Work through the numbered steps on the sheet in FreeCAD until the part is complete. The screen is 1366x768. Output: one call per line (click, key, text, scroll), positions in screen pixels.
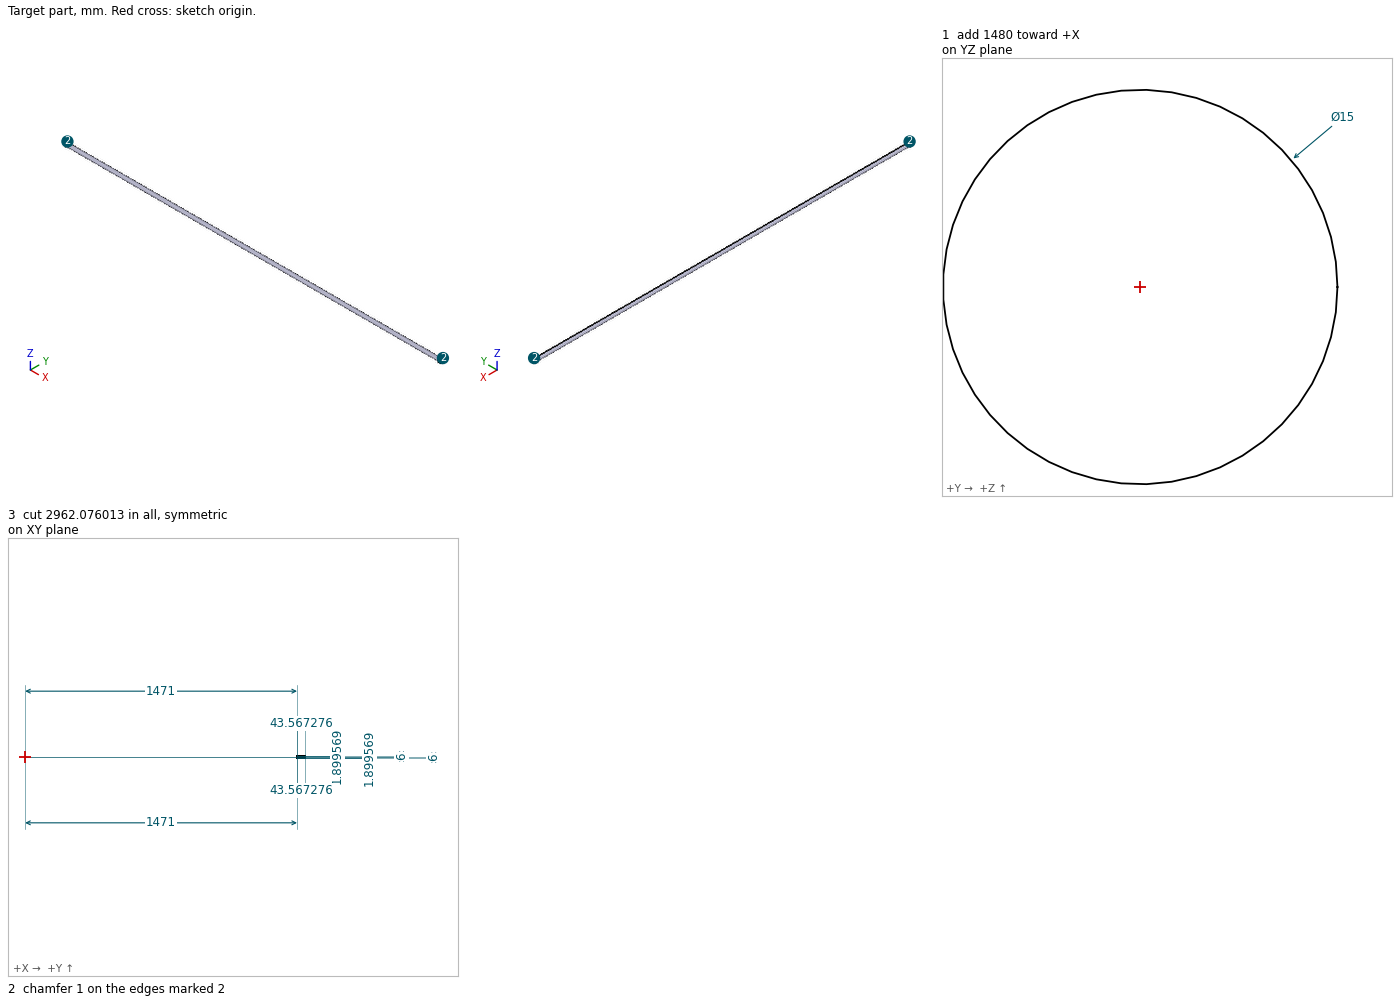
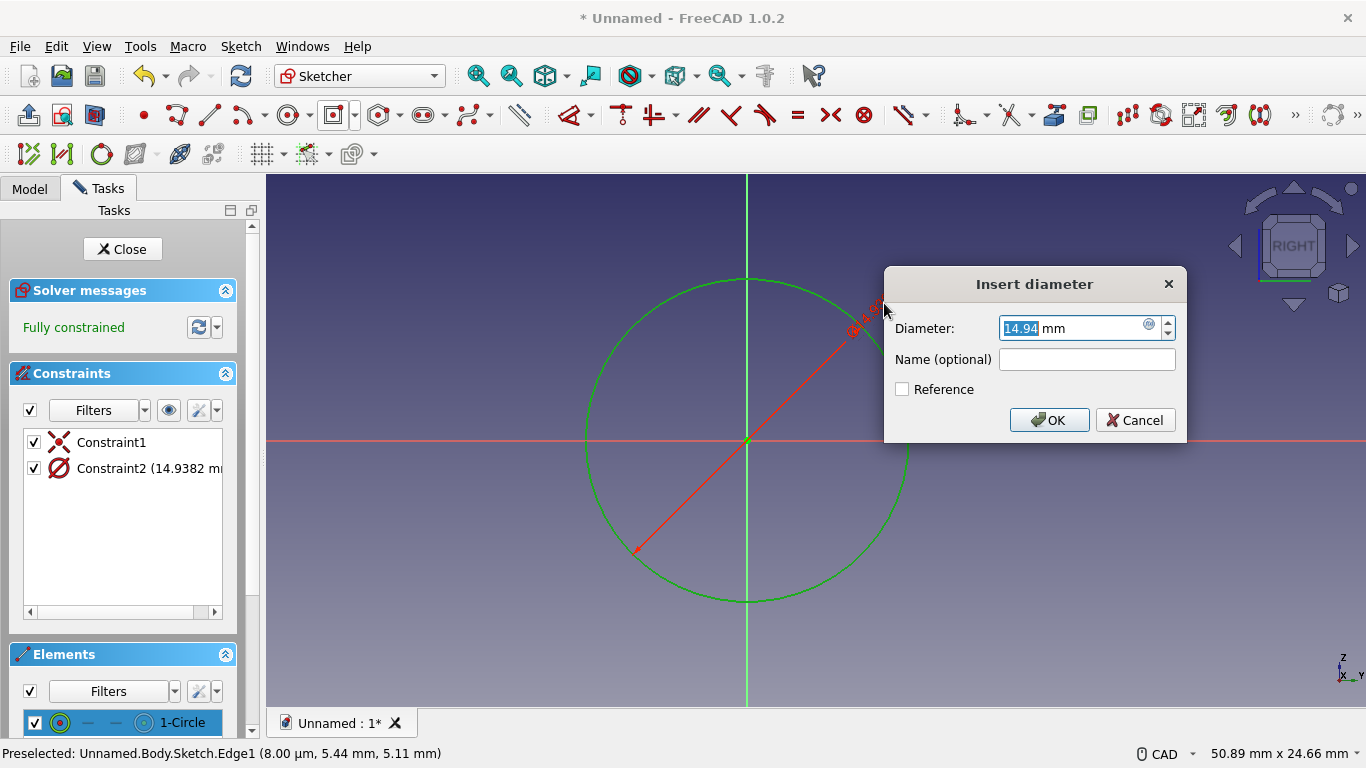
text(15)
key(Return)
key(Escape)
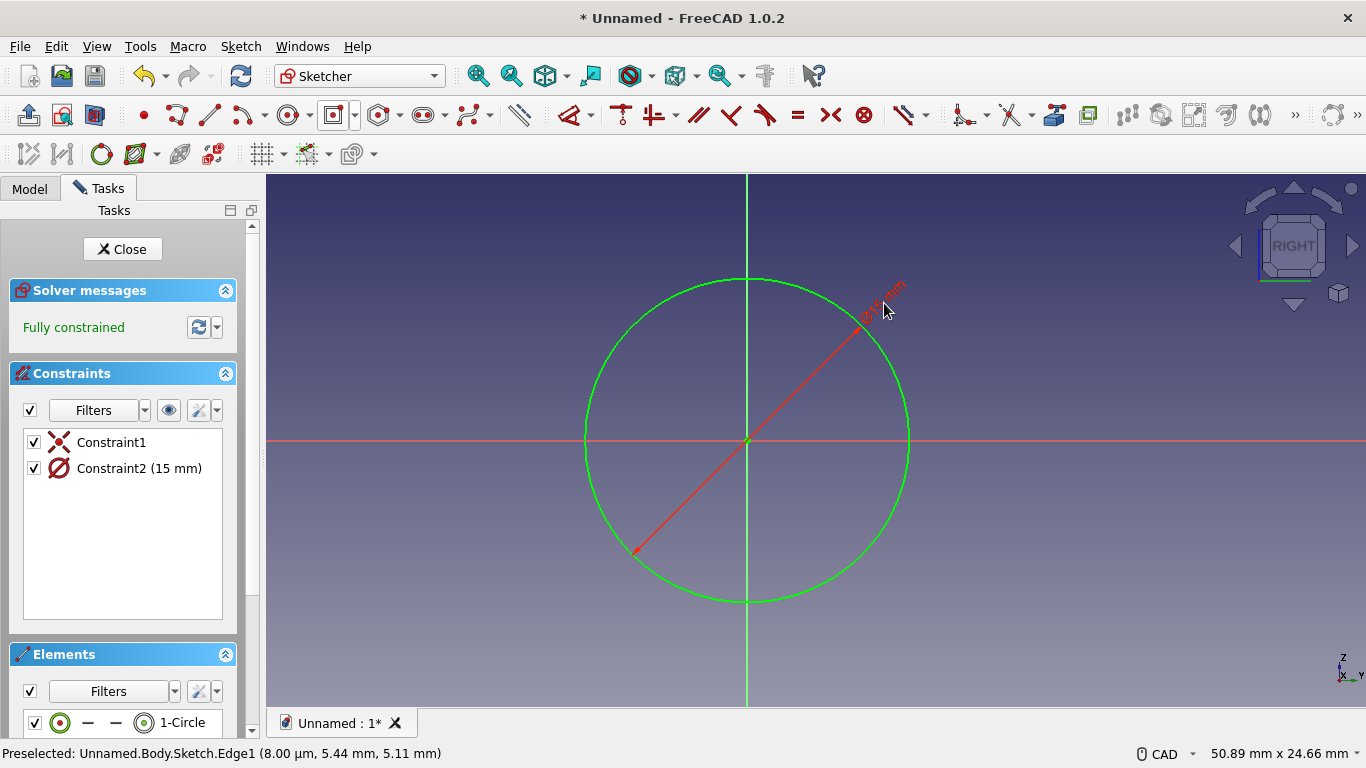
click(123, 249)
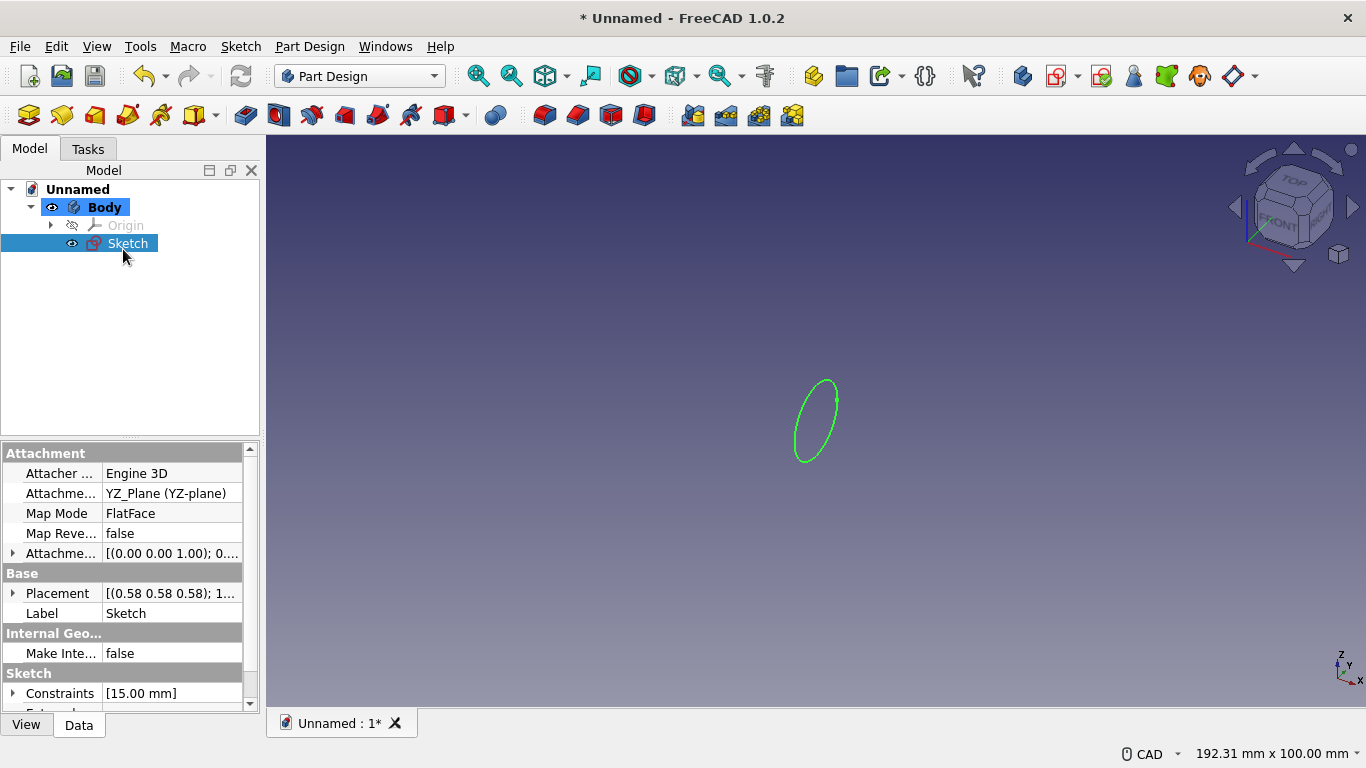
click(29, 116)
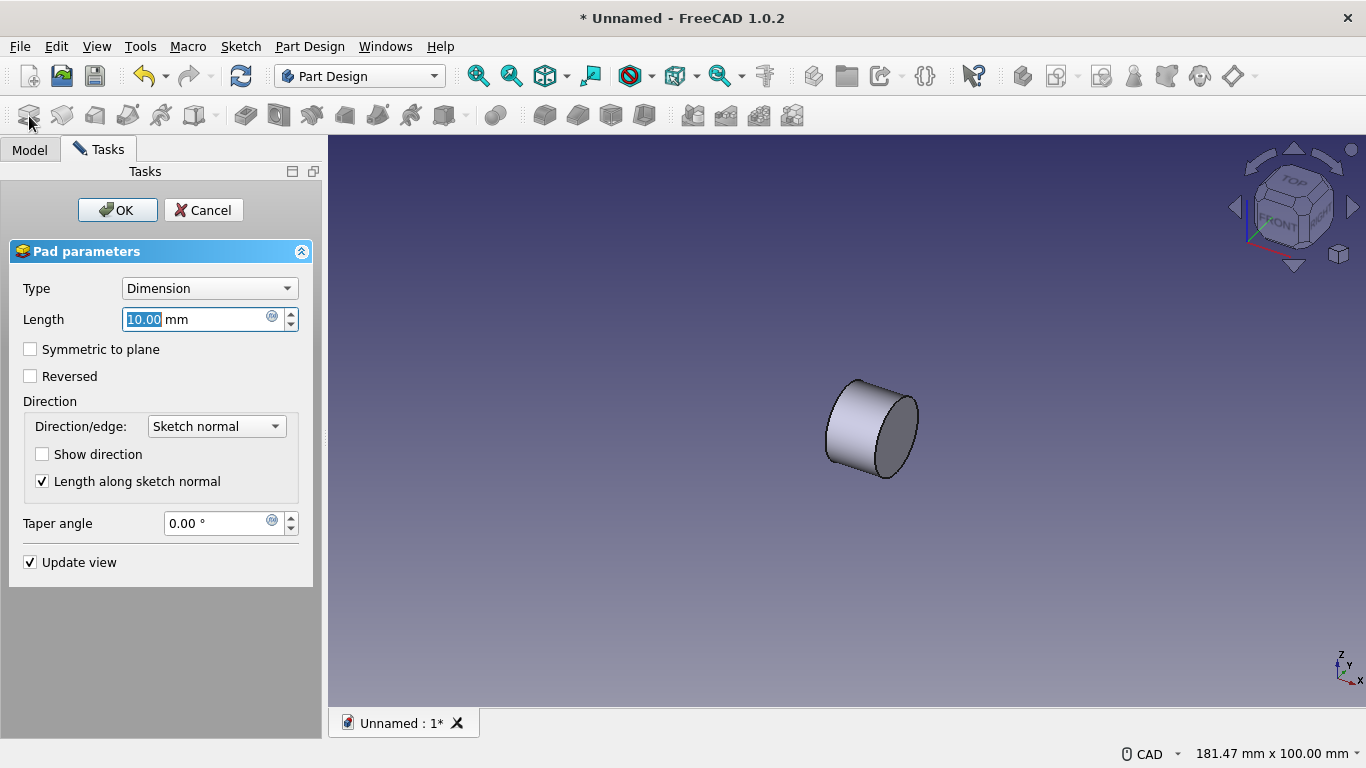
text(1480)
key(Tab)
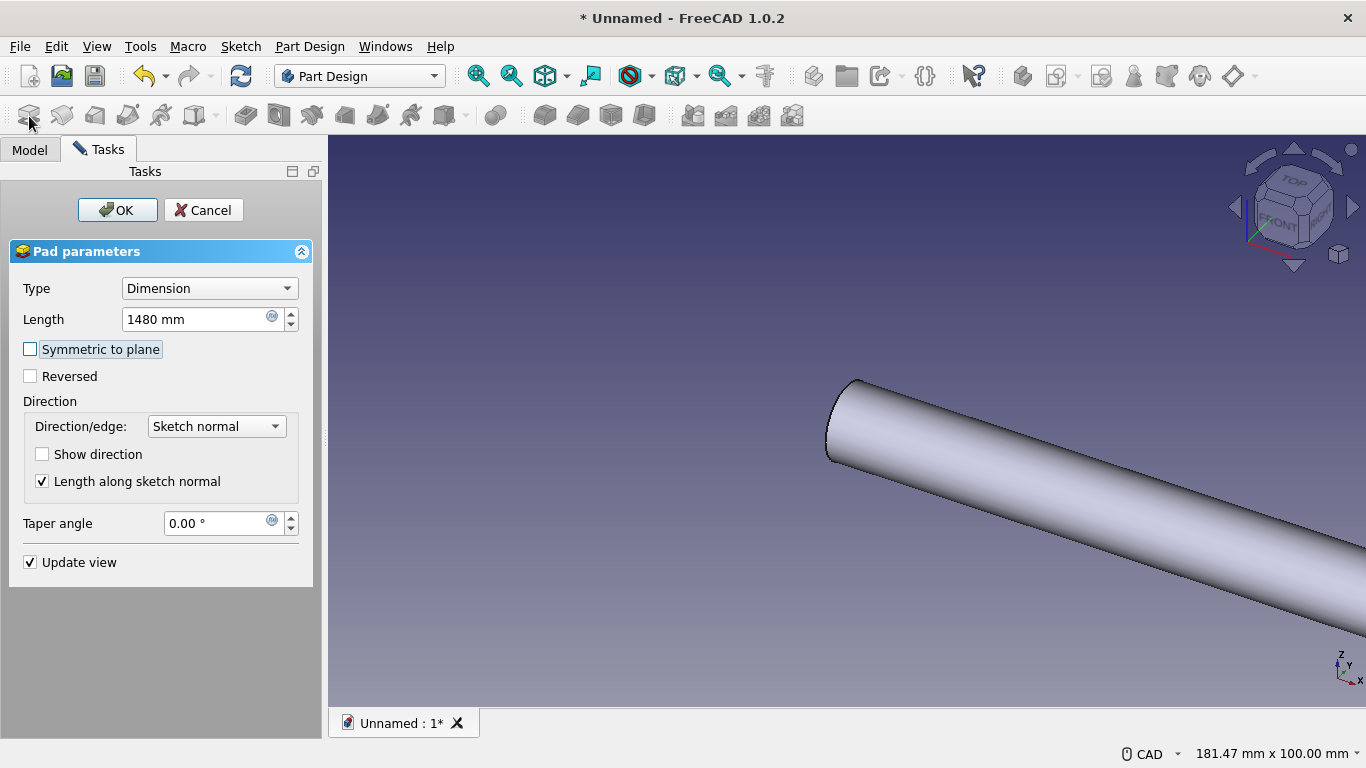
click(118, 210)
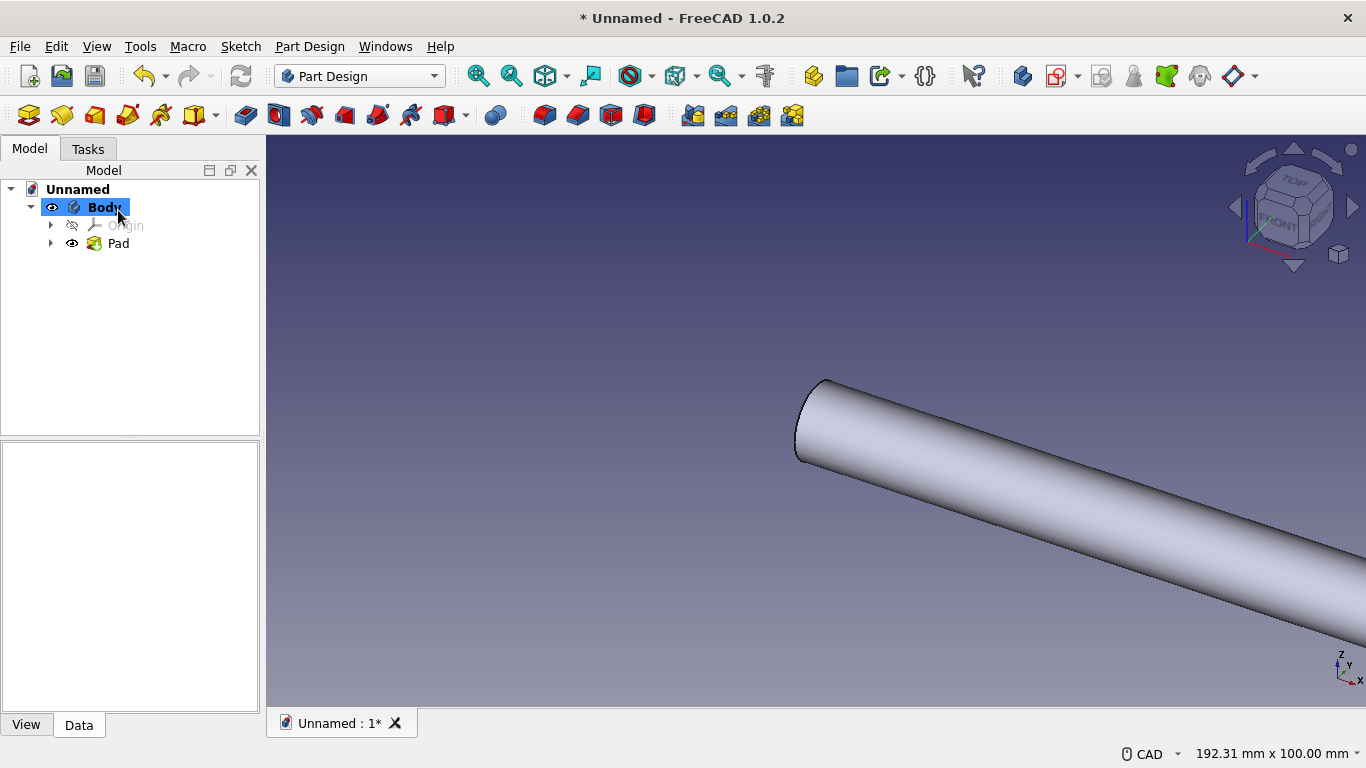
key(v)
key(f)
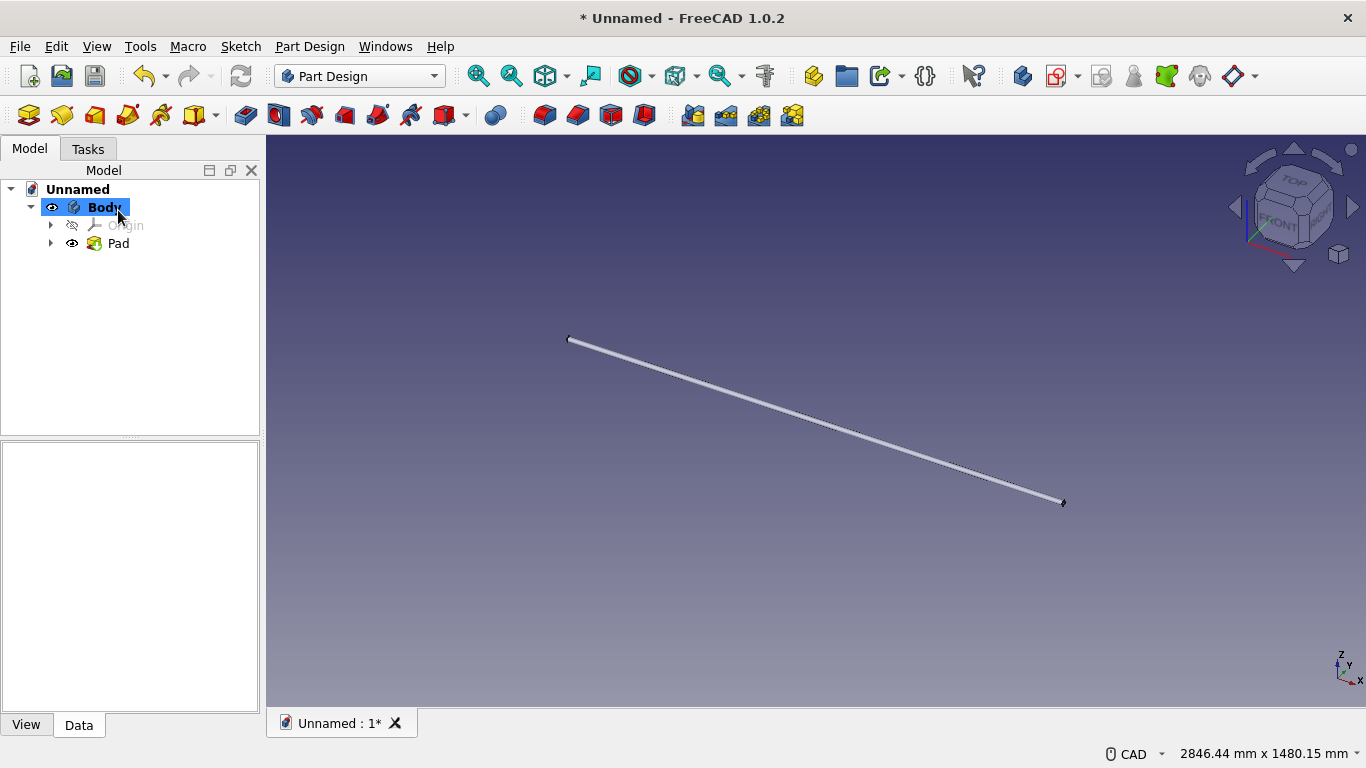
click(567, 341)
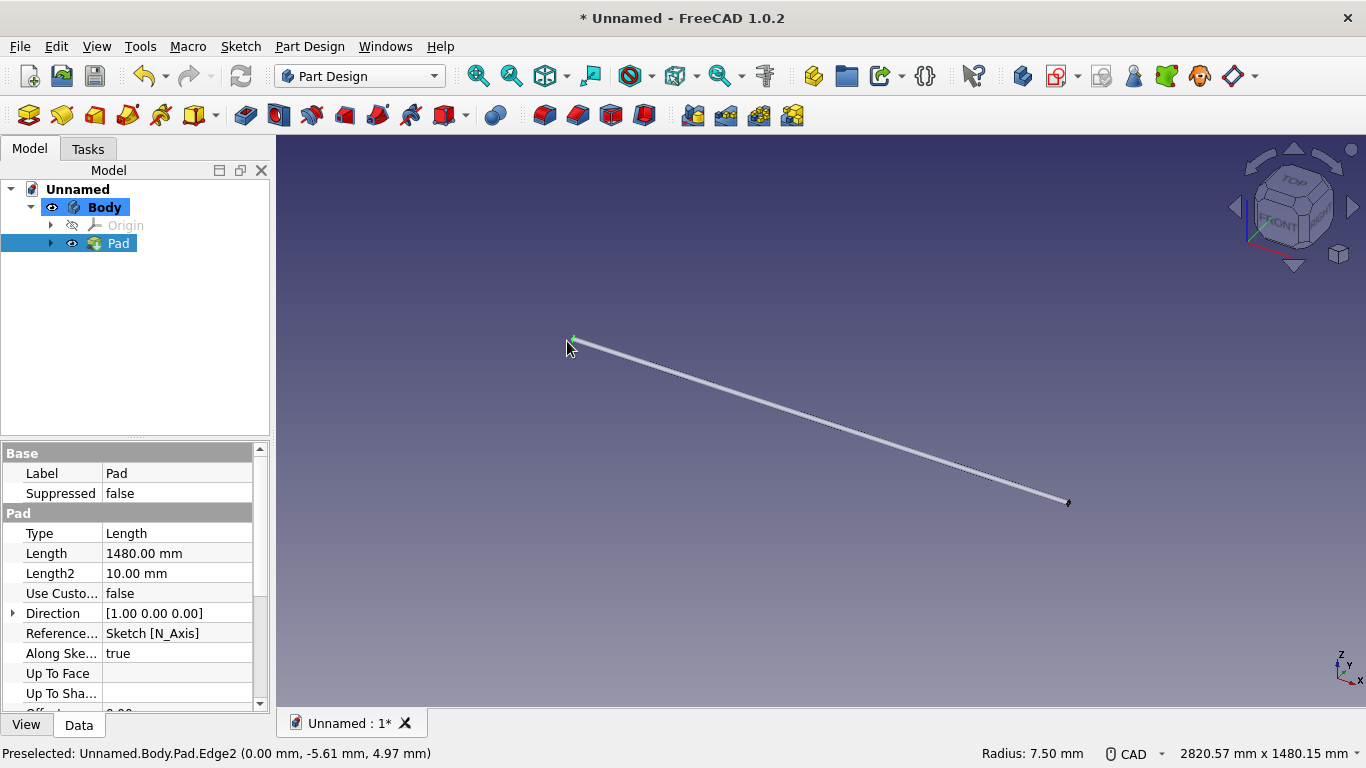
click(1067, 503, ctrl)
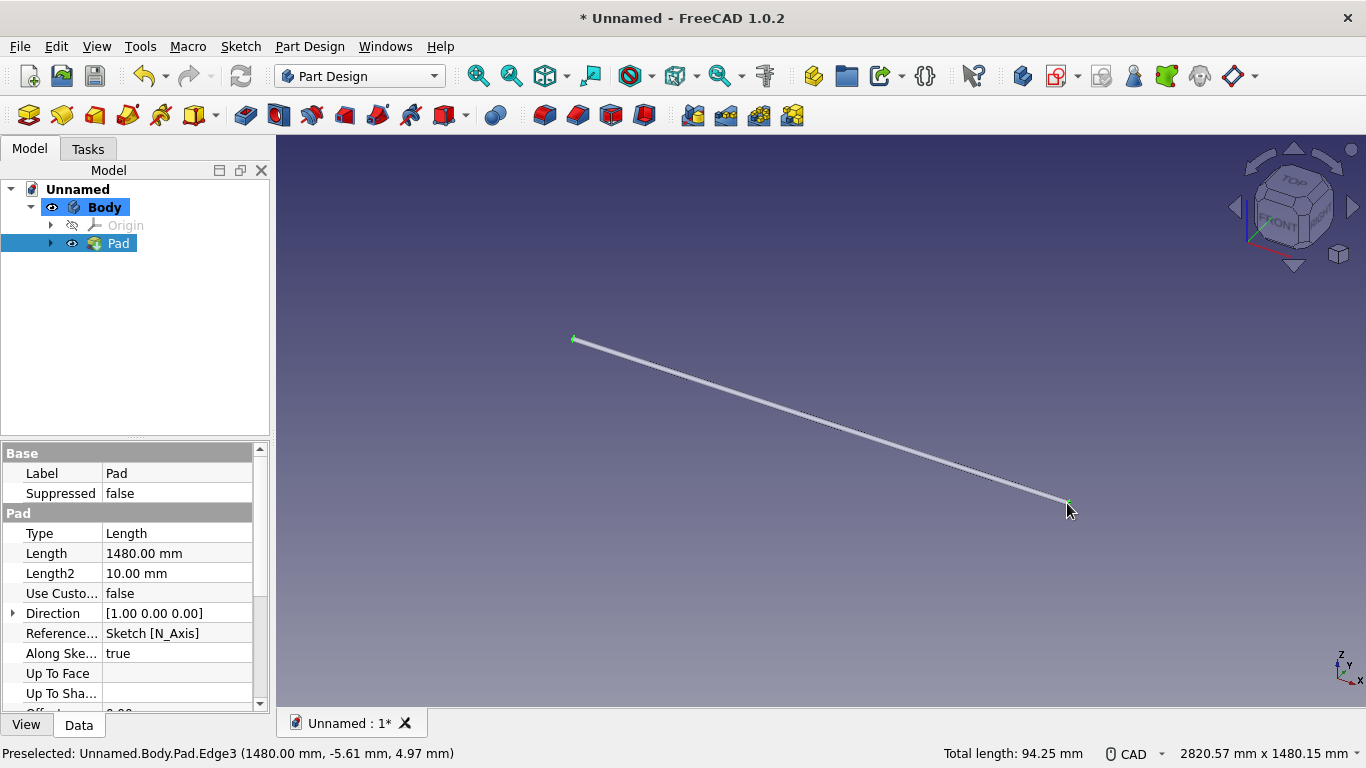
click(578, 116)